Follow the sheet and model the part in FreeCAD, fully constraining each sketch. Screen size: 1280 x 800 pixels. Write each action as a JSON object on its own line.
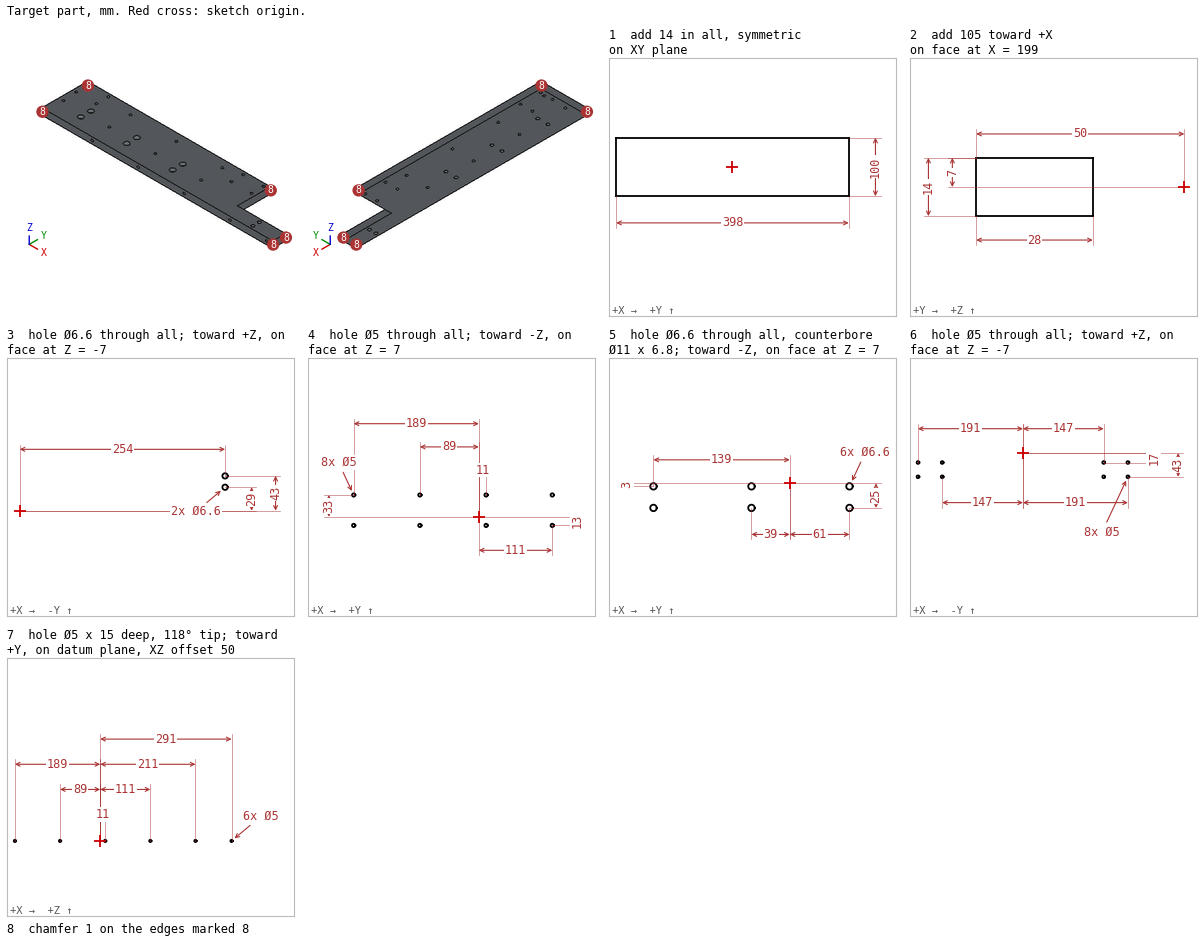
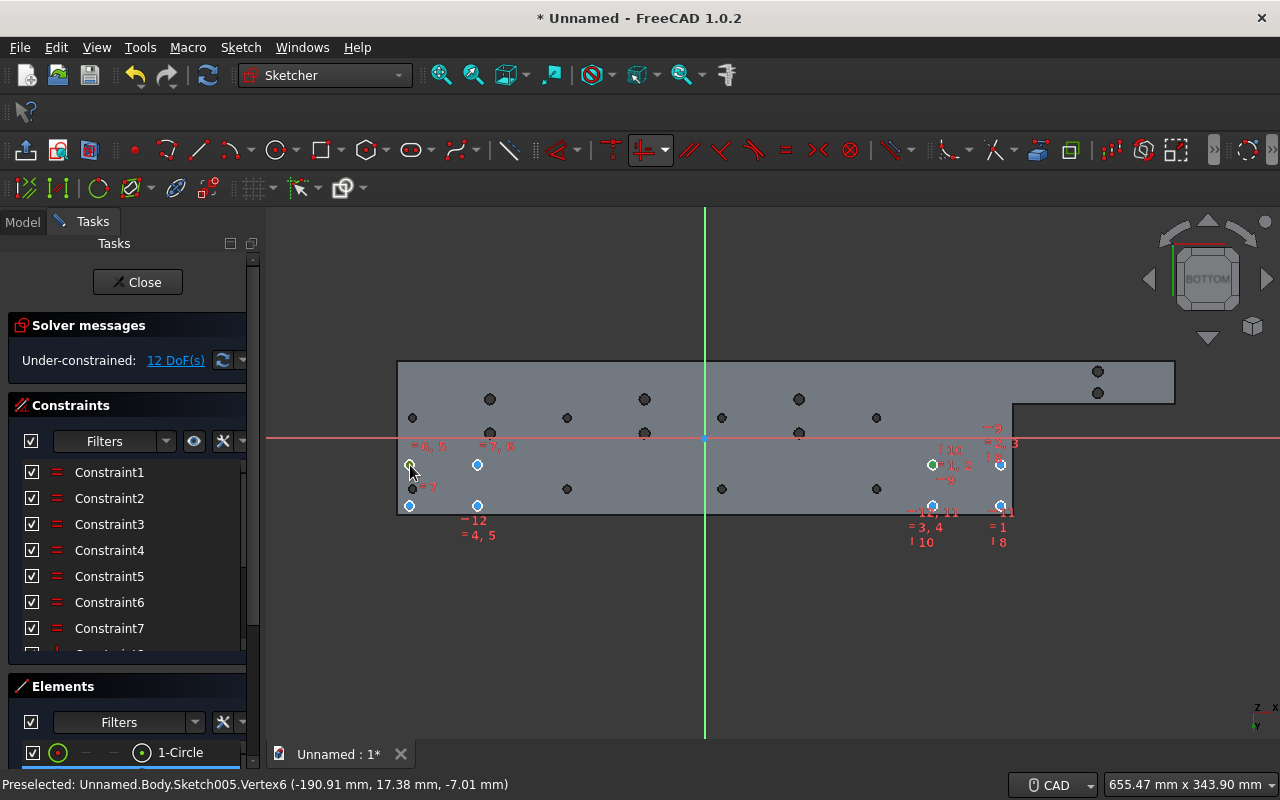
{"action": "key", "text": "h"}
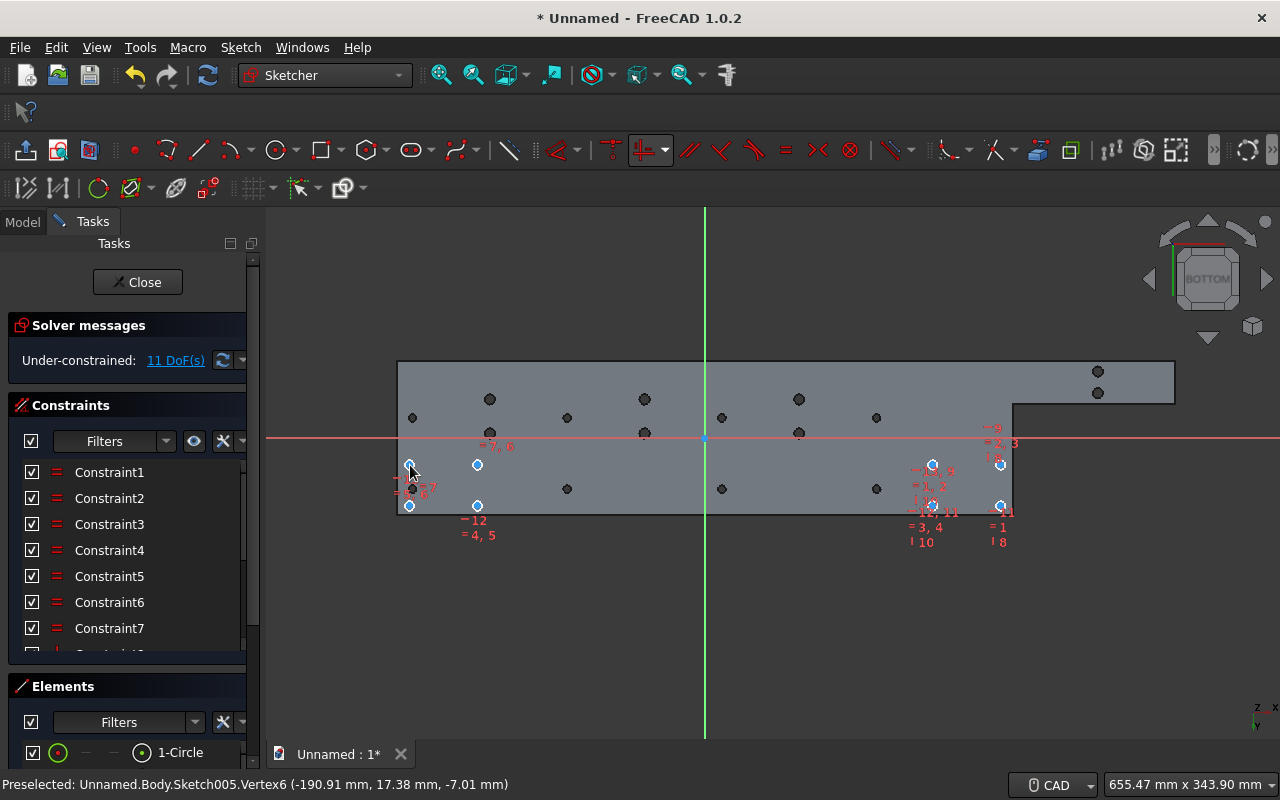
{"action": "left_click", "coordinate": [478, 506]}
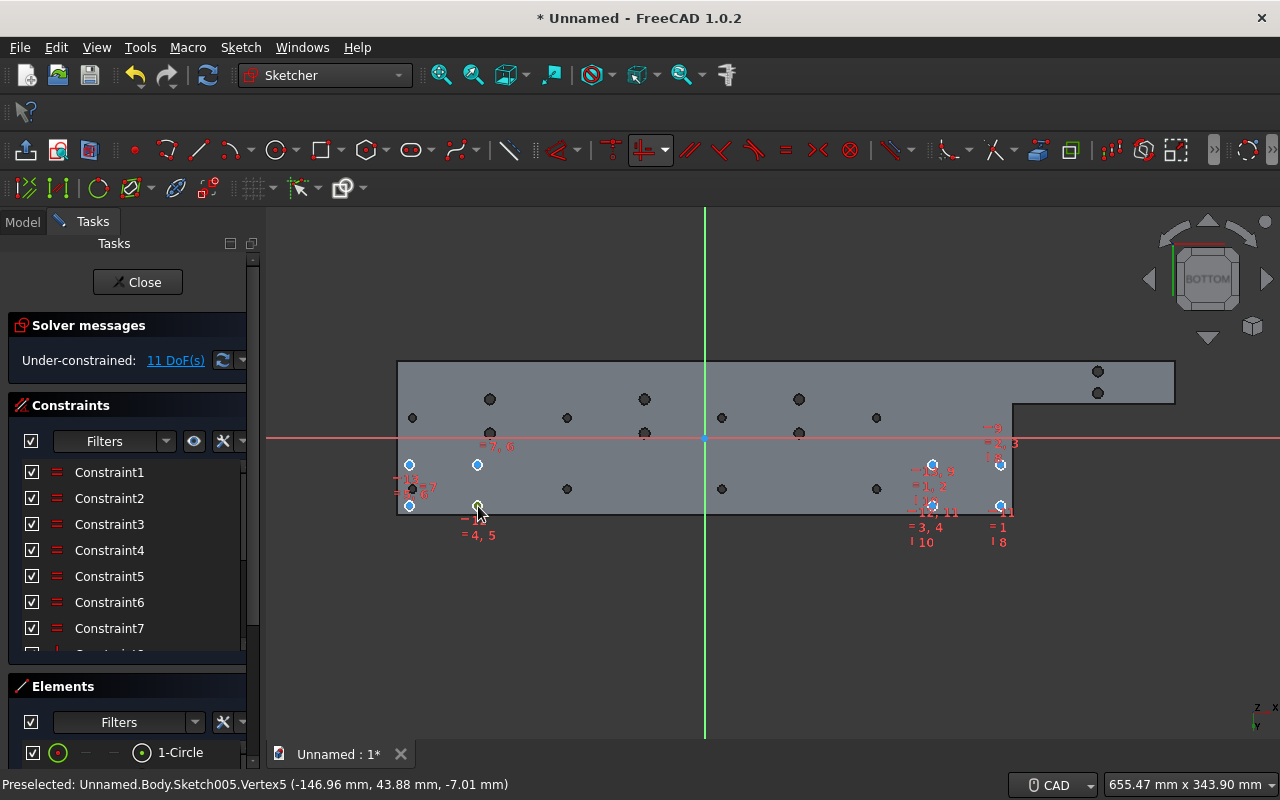
{"action": "left_click", "coordinate": [478, 465]}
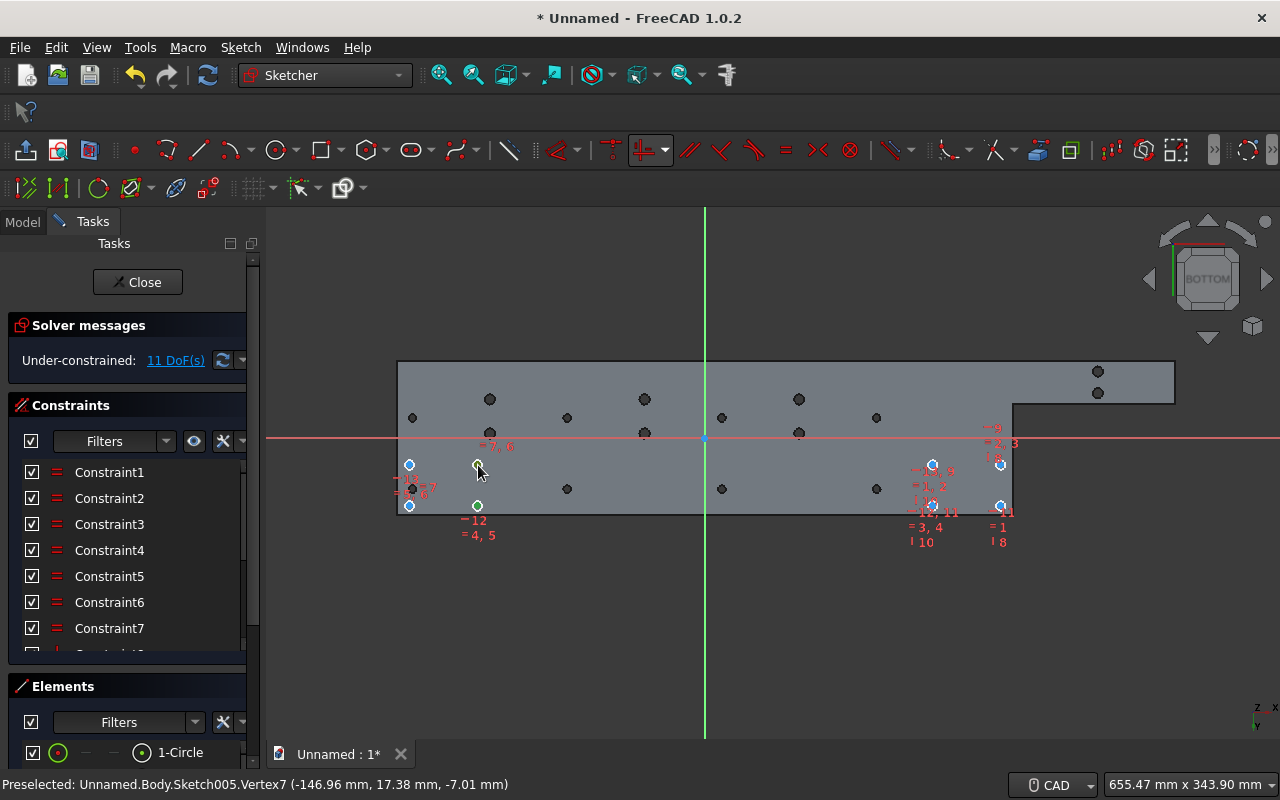
{"action": "key", "text": "v"}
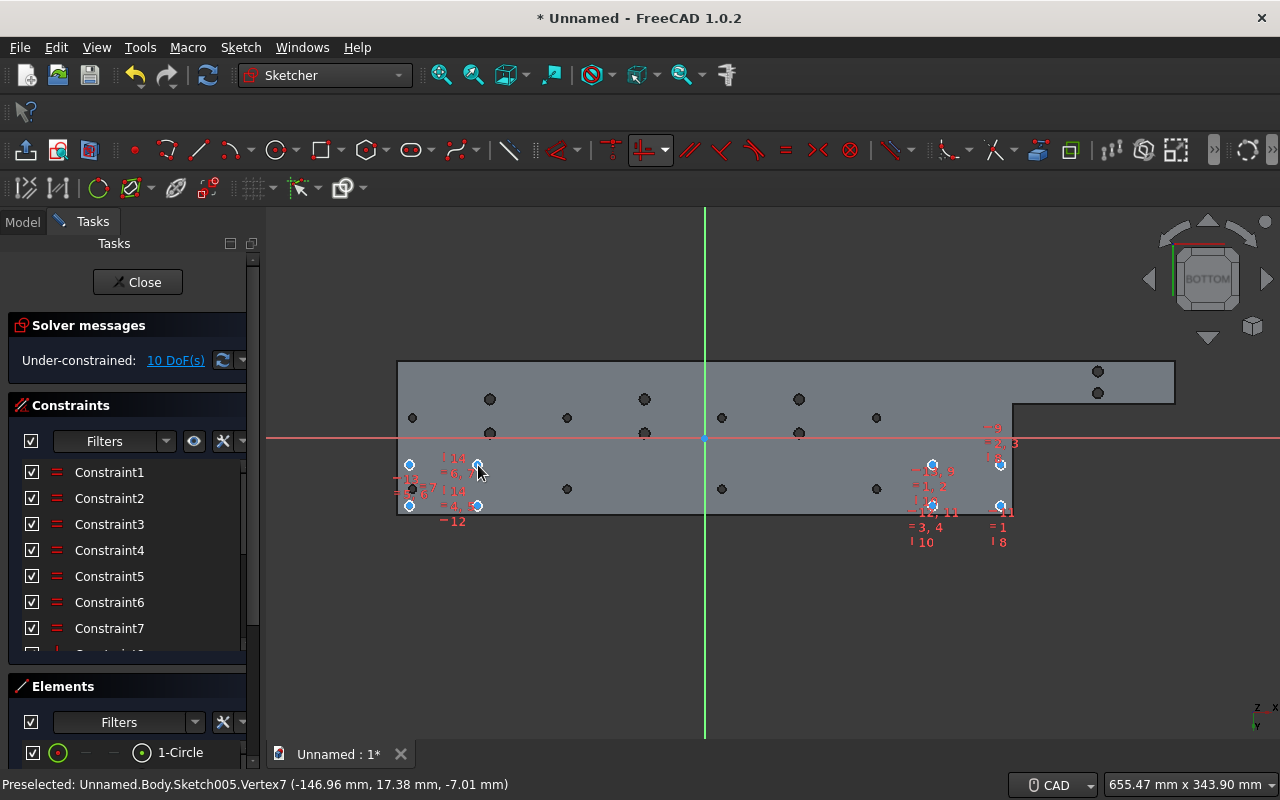
{"action": "left_click", "coordinate": [410, 465]}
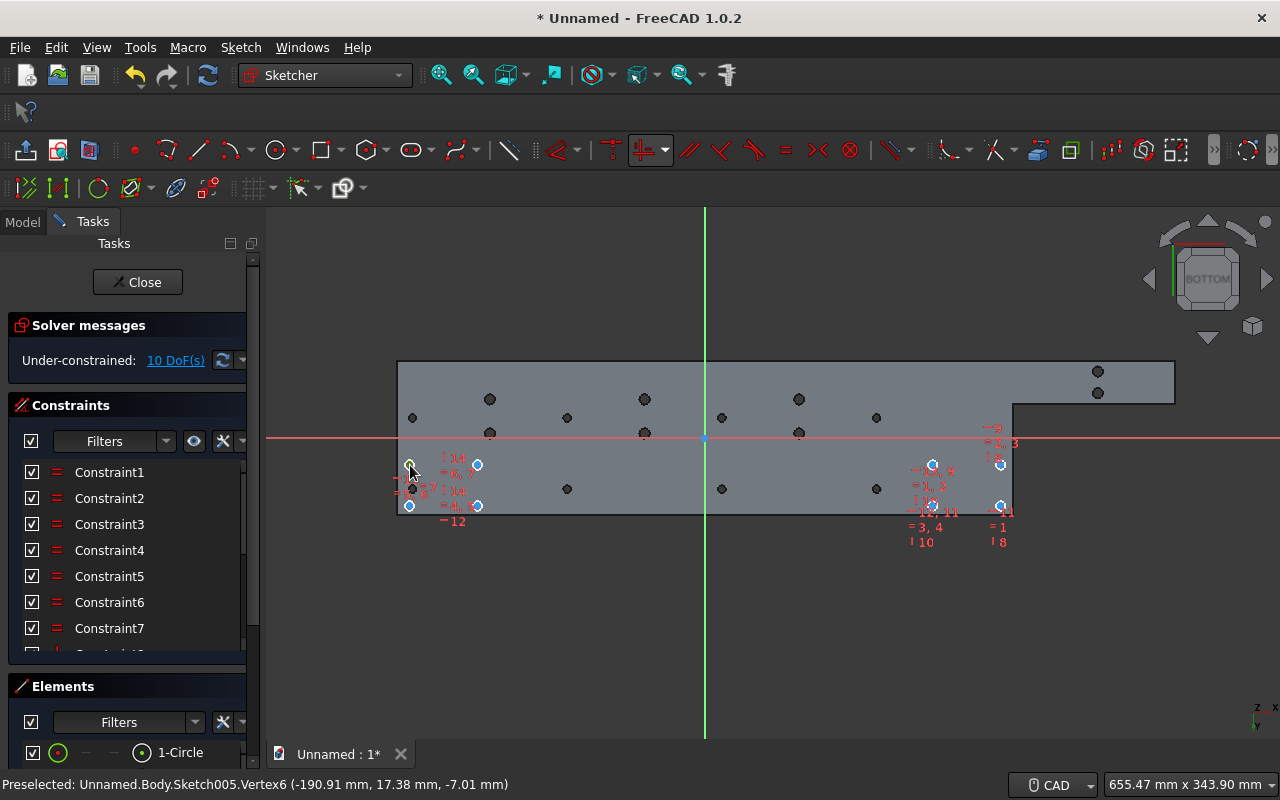
{"action": "left_click", "coordinate": [478, 465]}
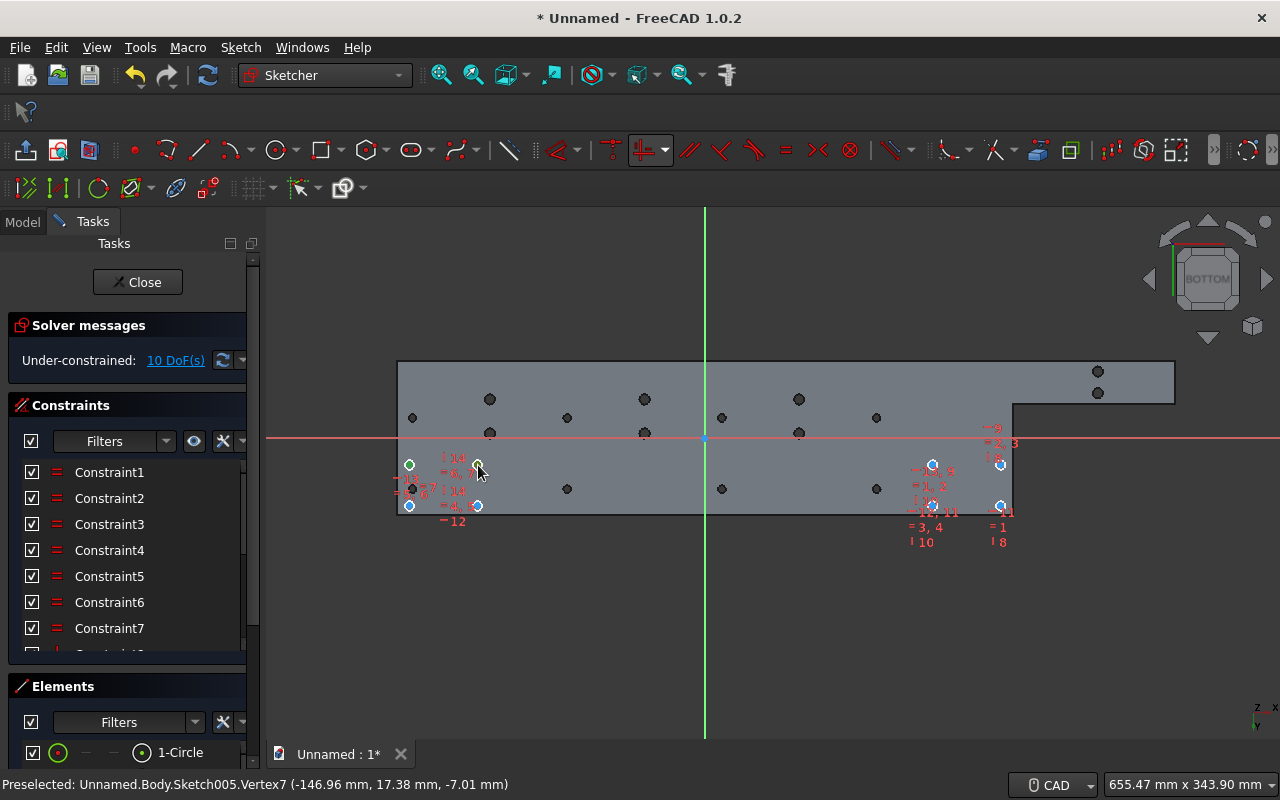
{"action": "key", "text": "h"}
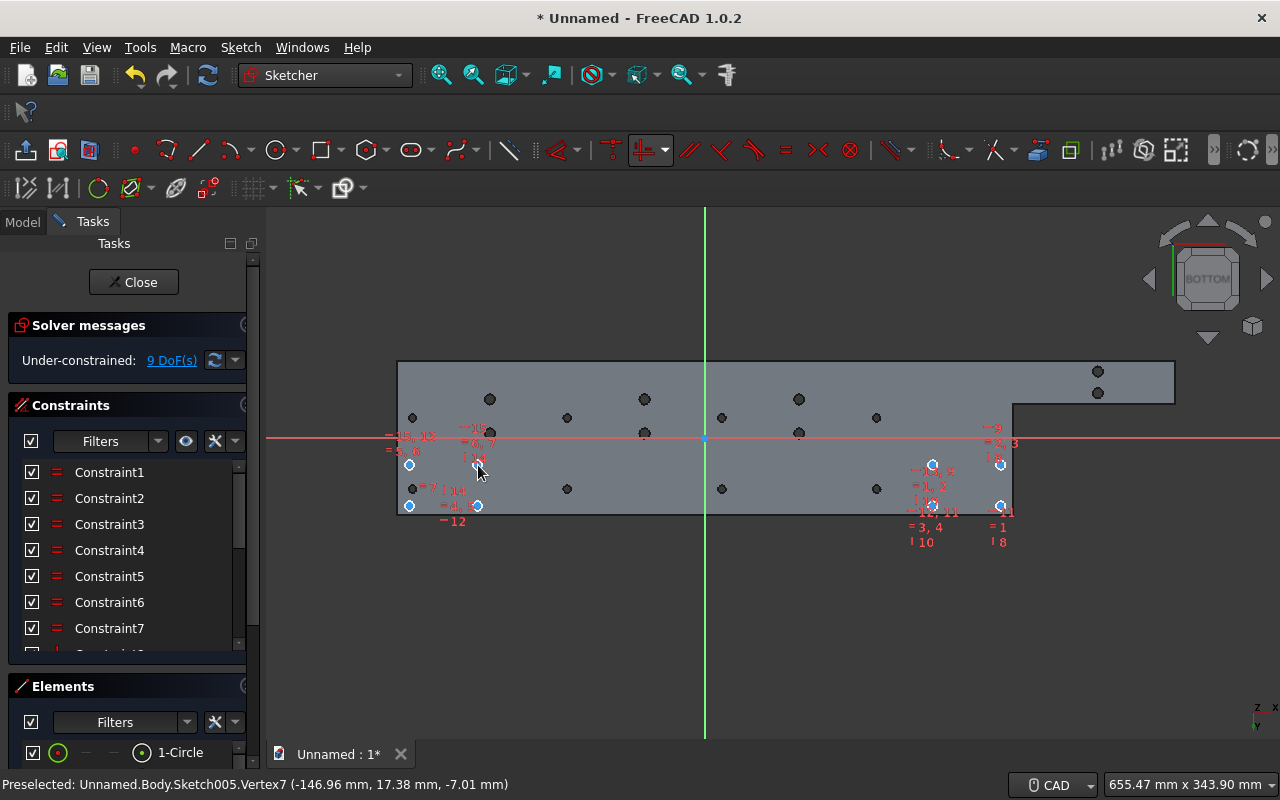
{"action": "left_click", "coordinate": [410, 465]}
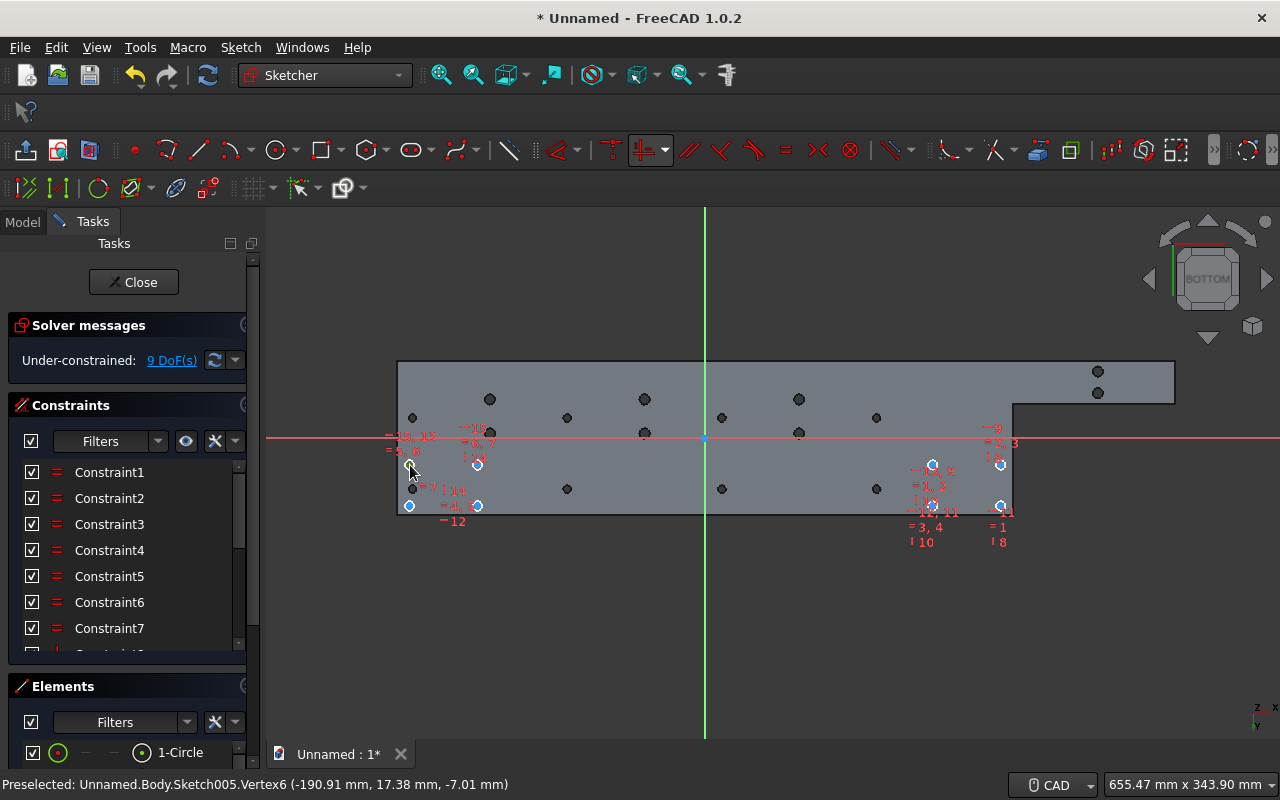
{"action": "left_click", "coordinate": [410, 506]}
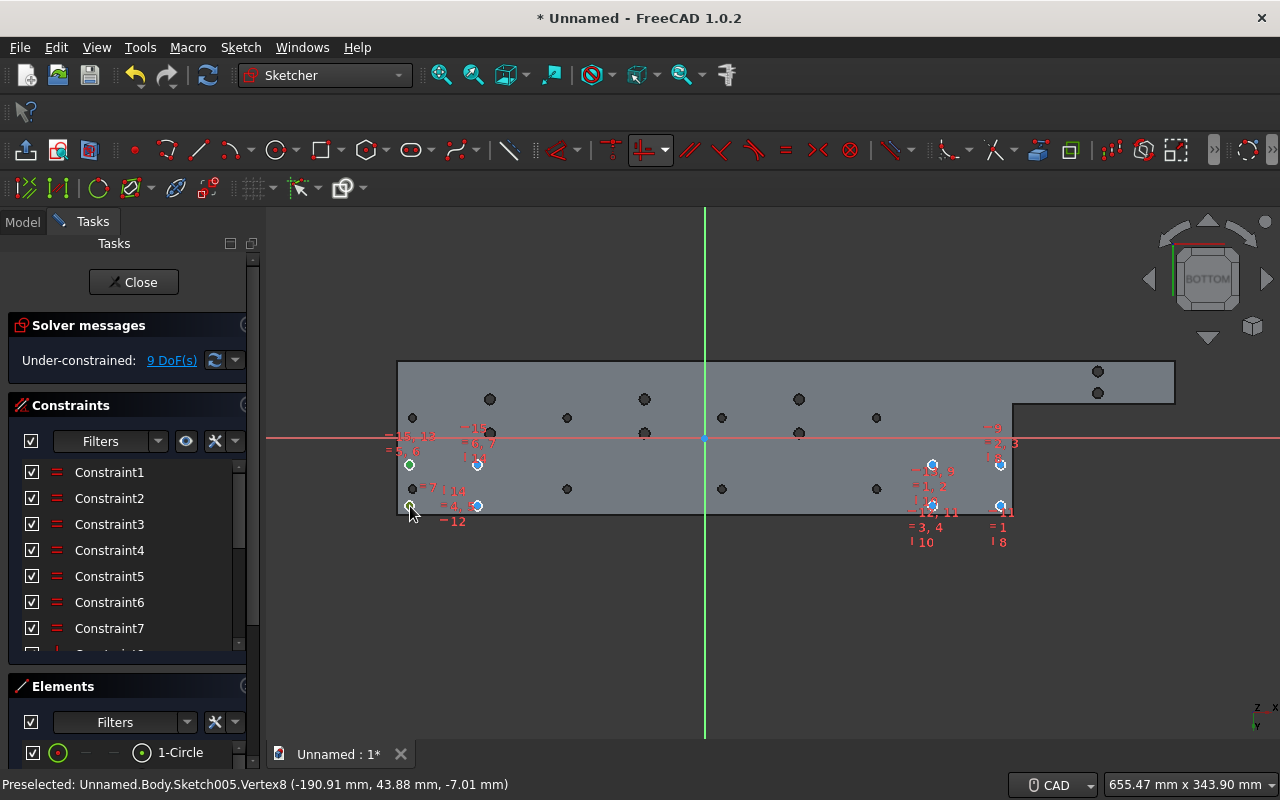
{"action": "left_click", "coordinate": [668, 150]}